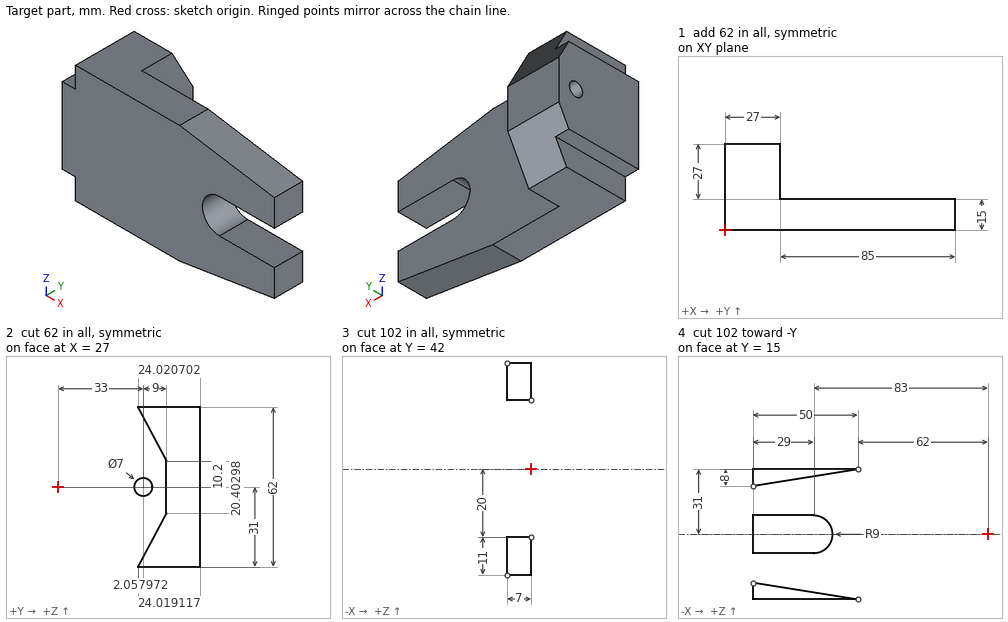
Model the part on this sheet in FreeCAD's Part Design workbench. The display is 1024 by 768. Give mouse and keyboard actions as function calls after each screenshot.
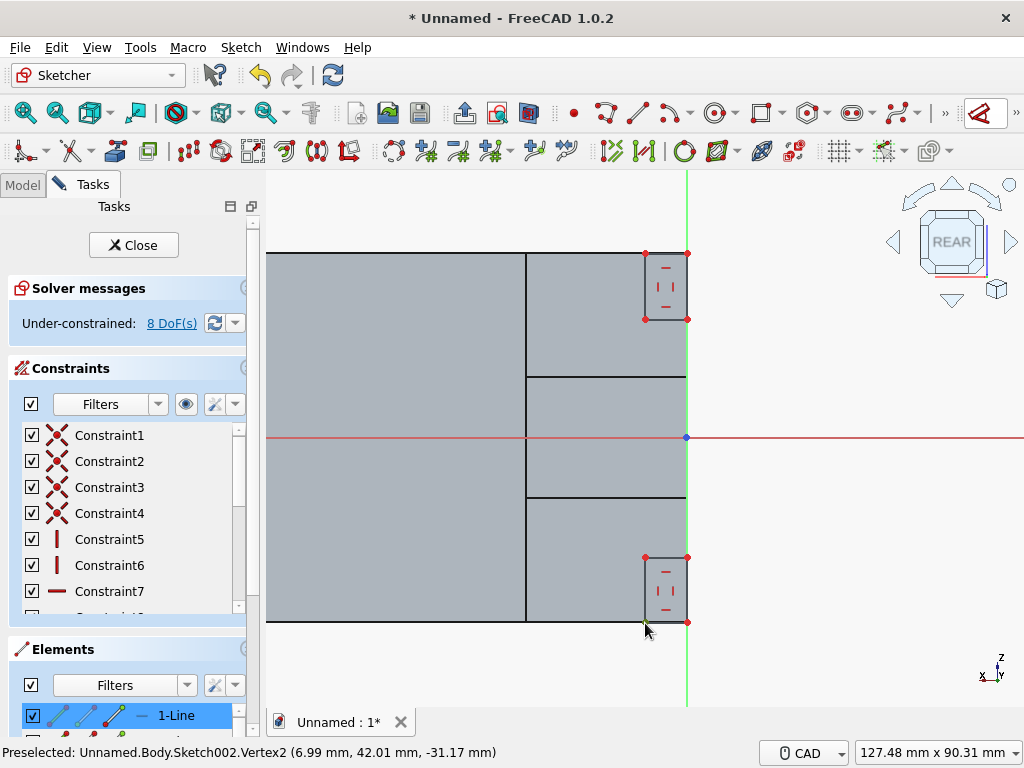
click(645, 254)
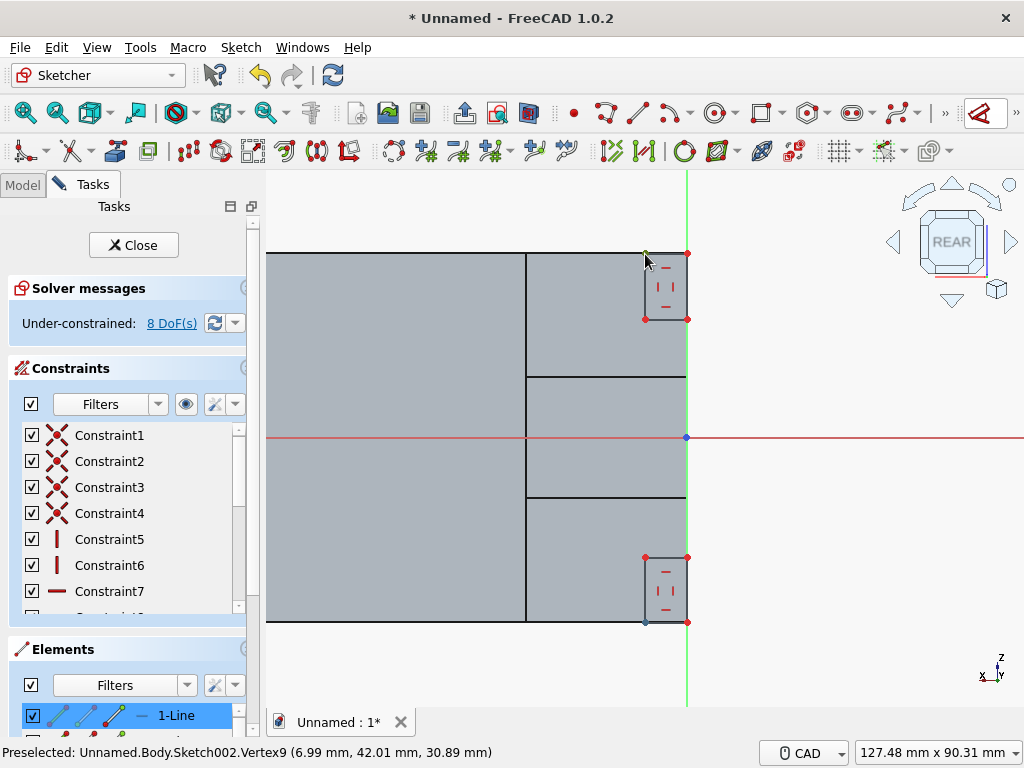
click(334, 438)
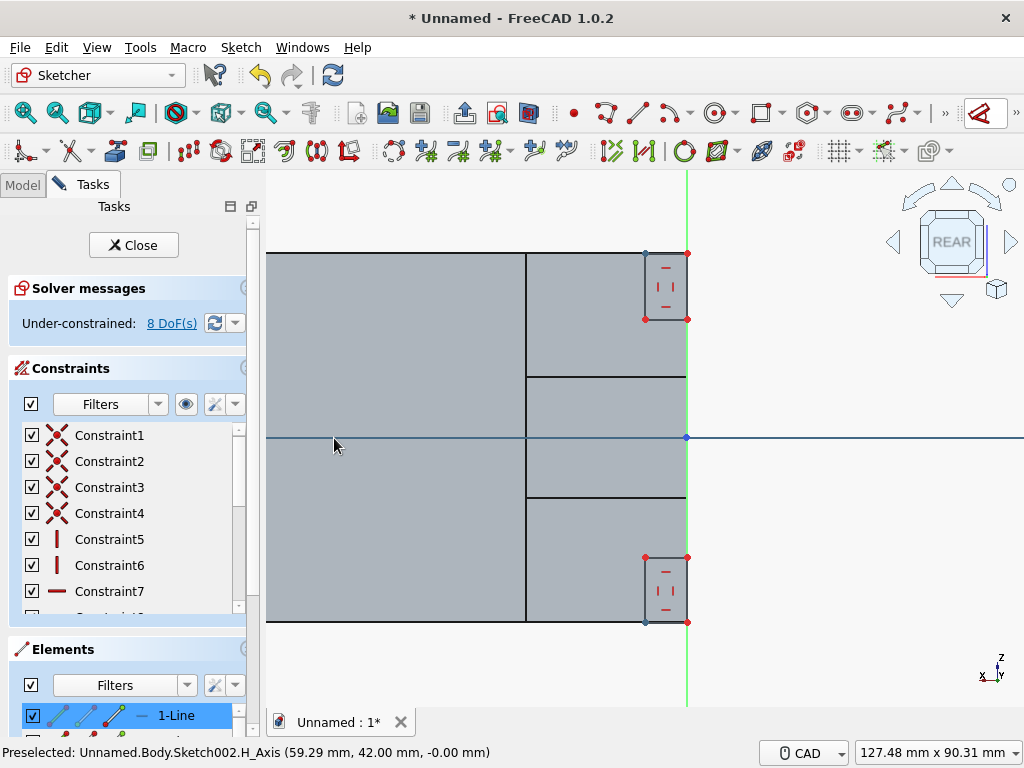
key(s)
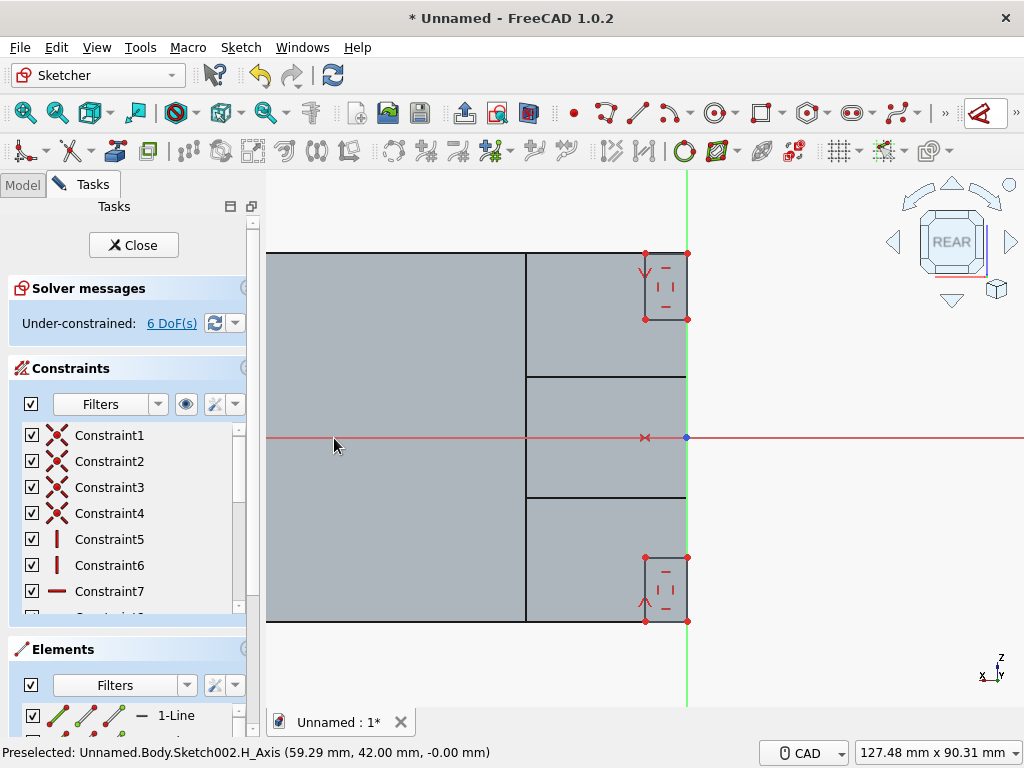
click(687, 558)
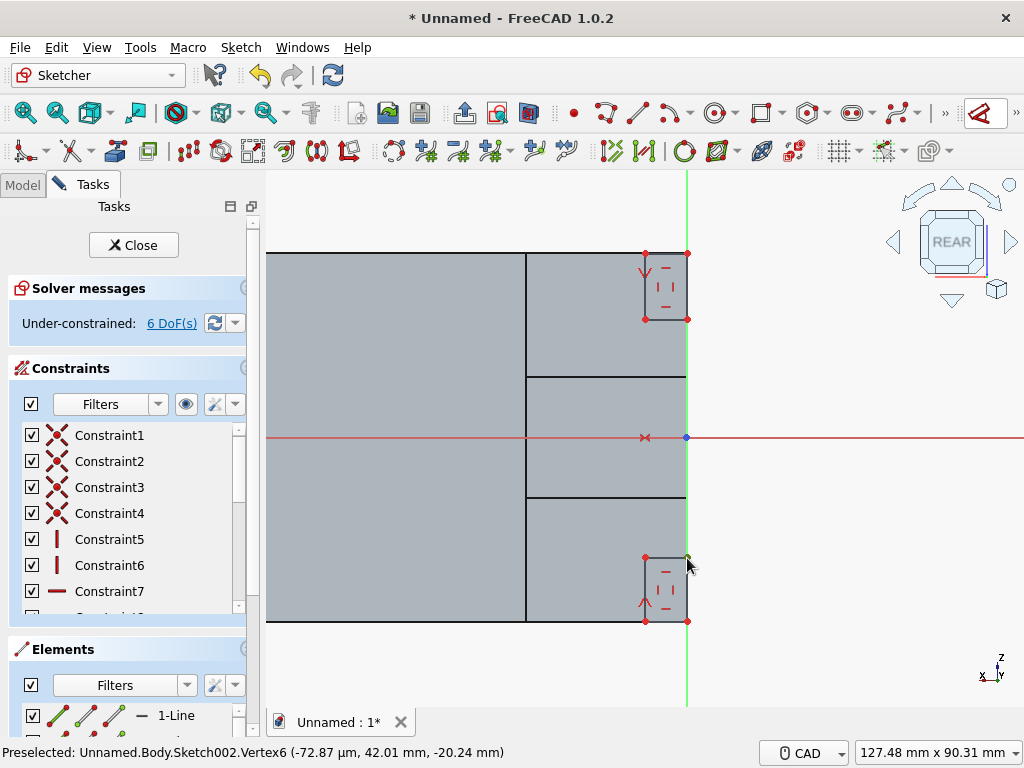
click(687, 320)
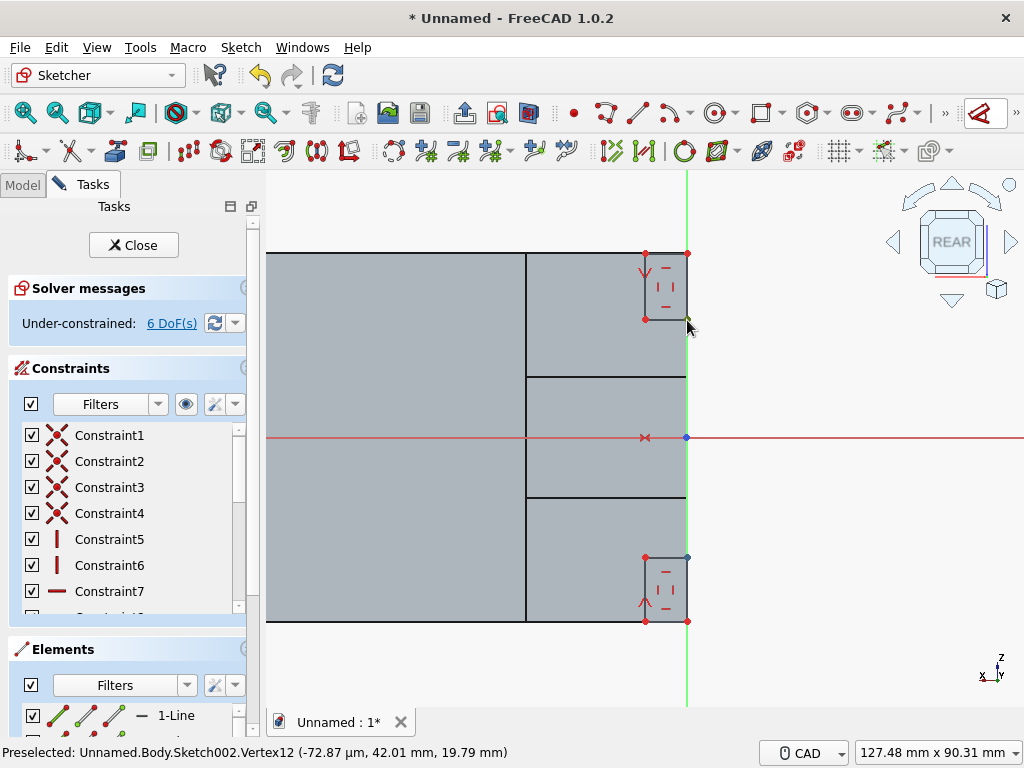
click(334, 438)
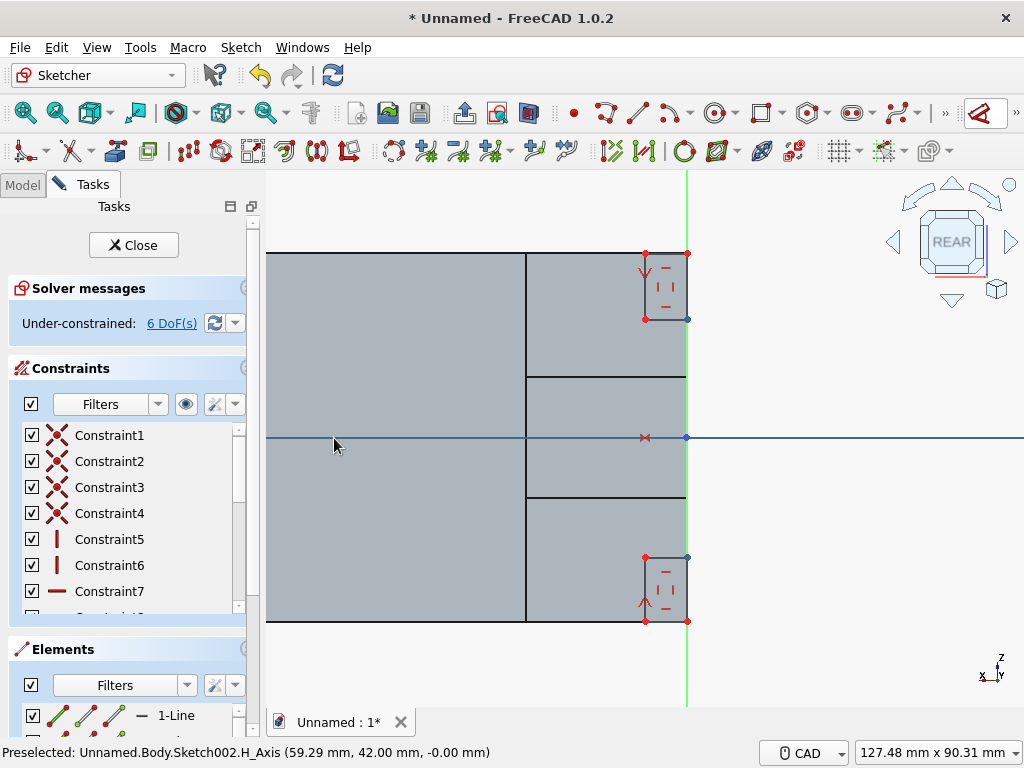
key(s)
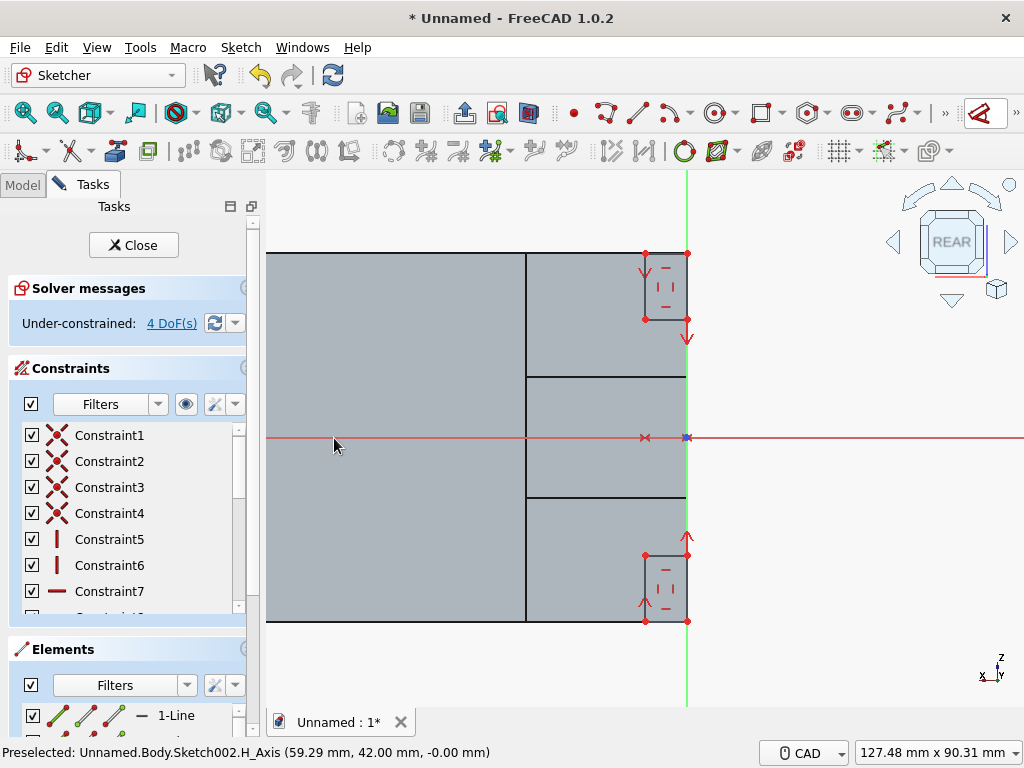
click(687, 622)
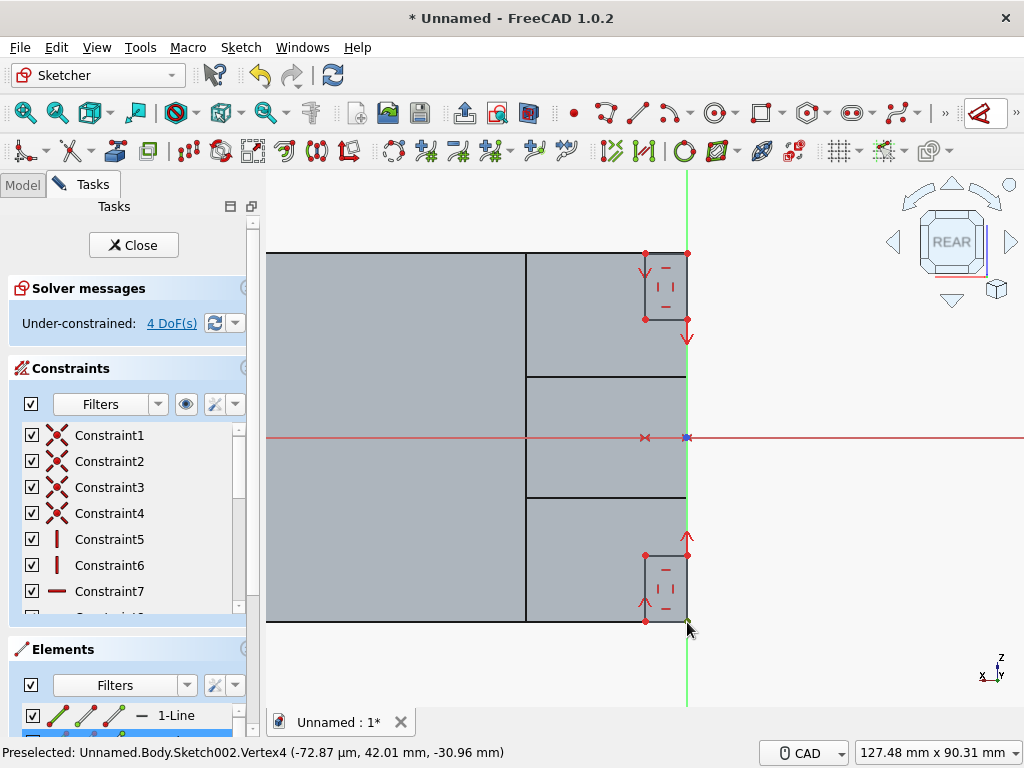
click(687, 507)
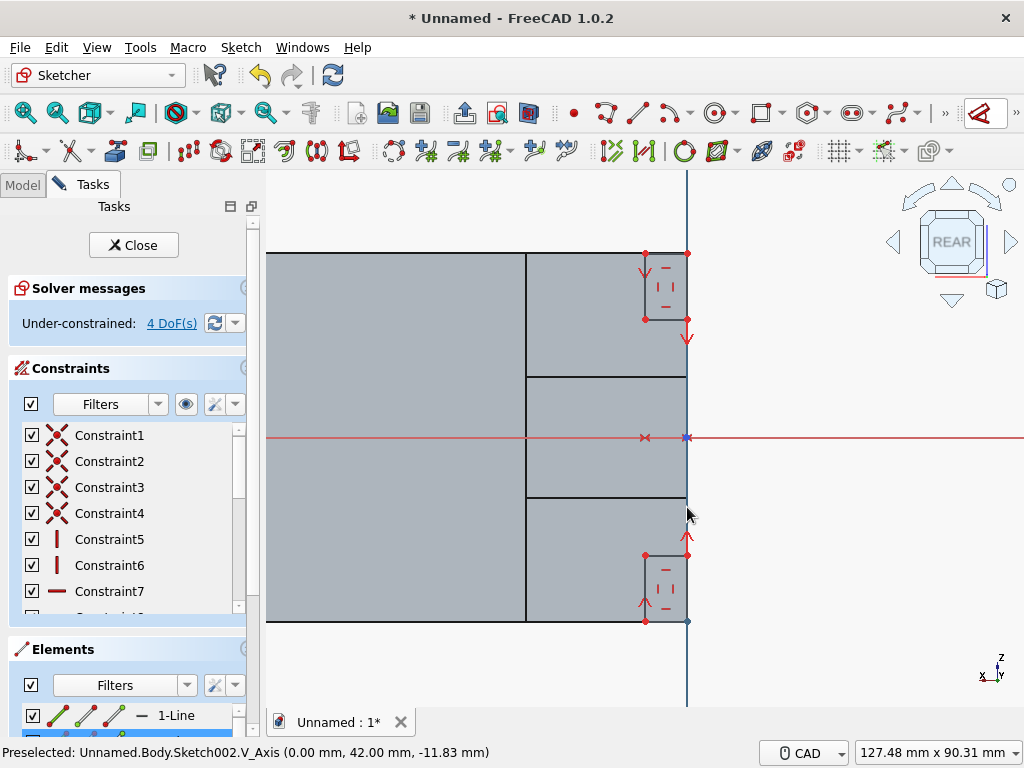
key(c)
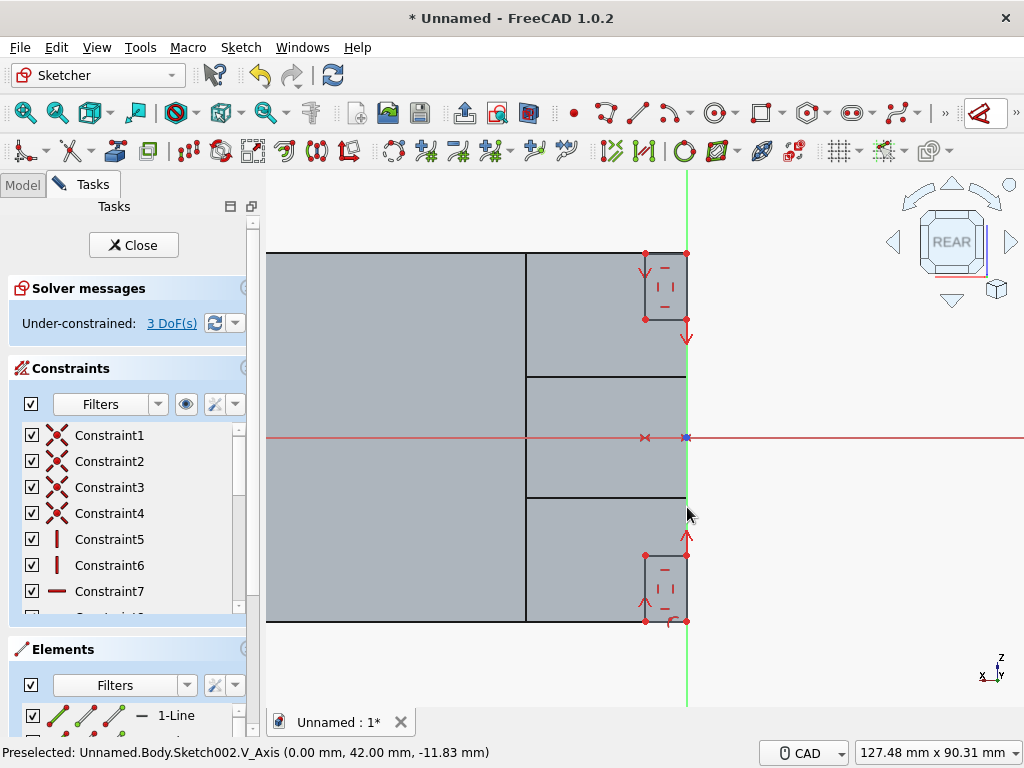
click(657, 622)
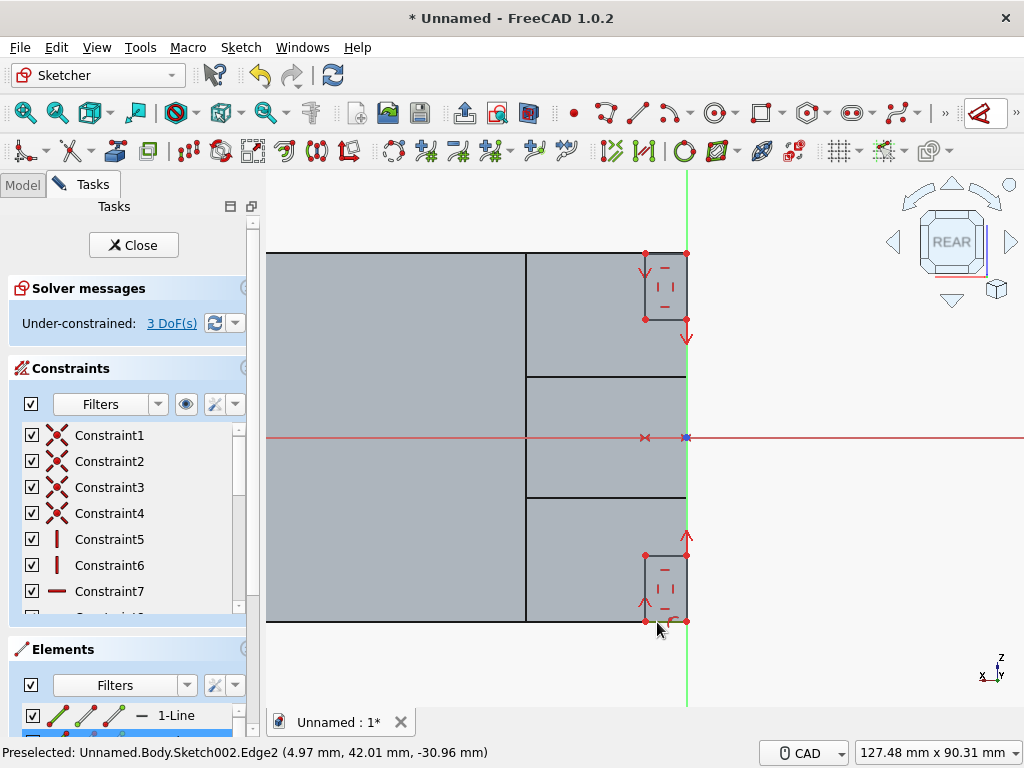
click(1002, 114)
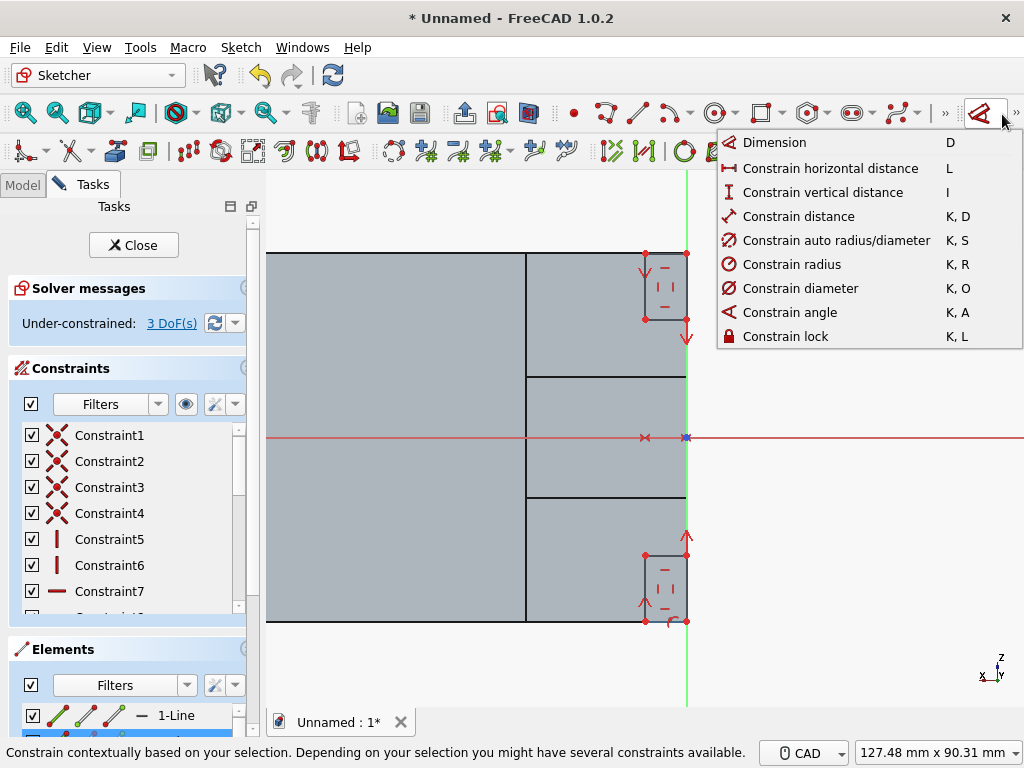
click(870, 168)